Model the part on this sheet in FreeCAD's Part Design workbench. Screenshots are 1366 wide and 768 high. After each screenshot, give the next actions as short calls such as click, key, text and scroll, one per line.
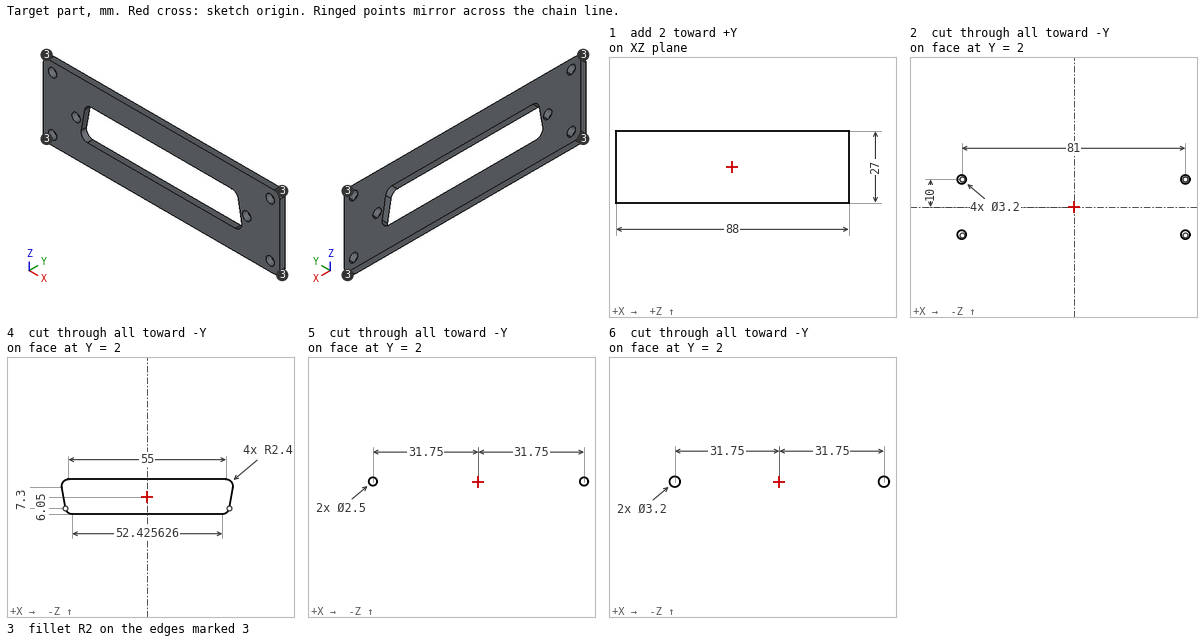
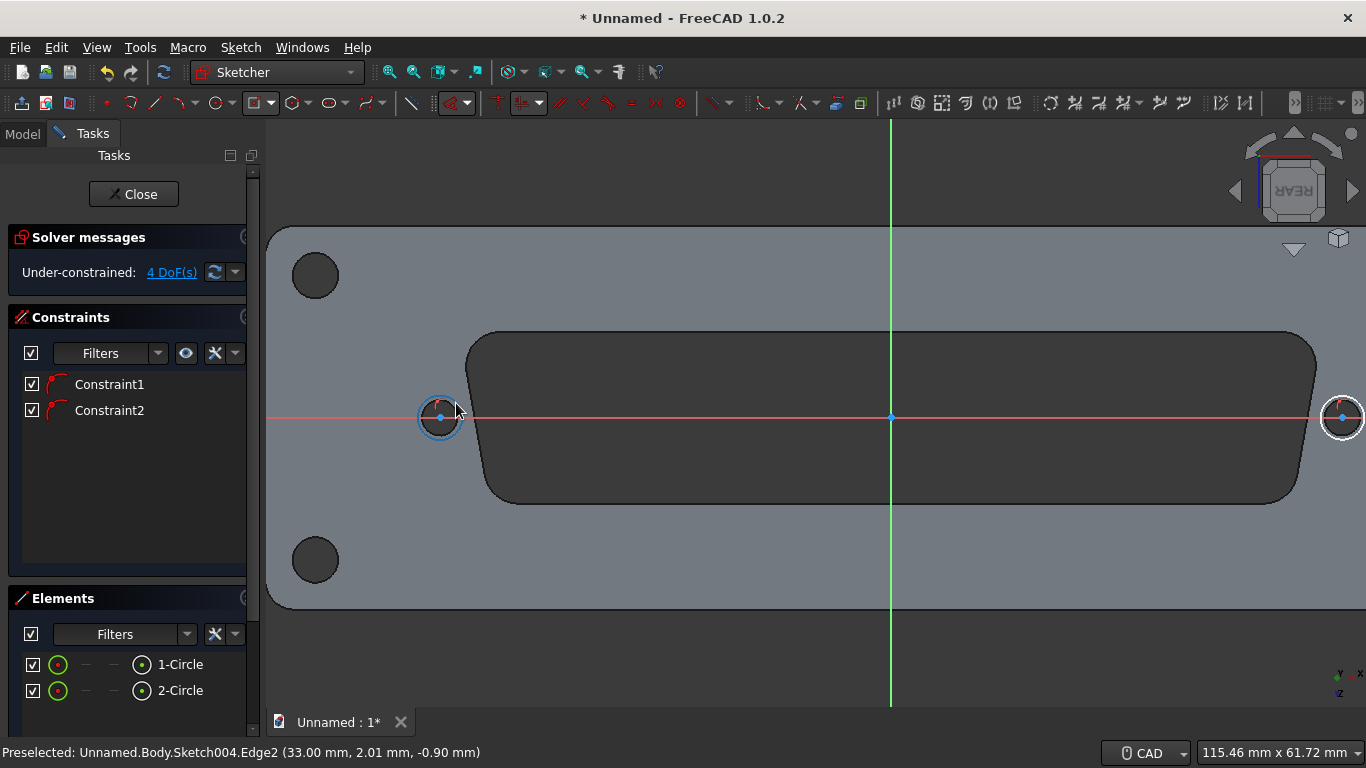
click(456, 402)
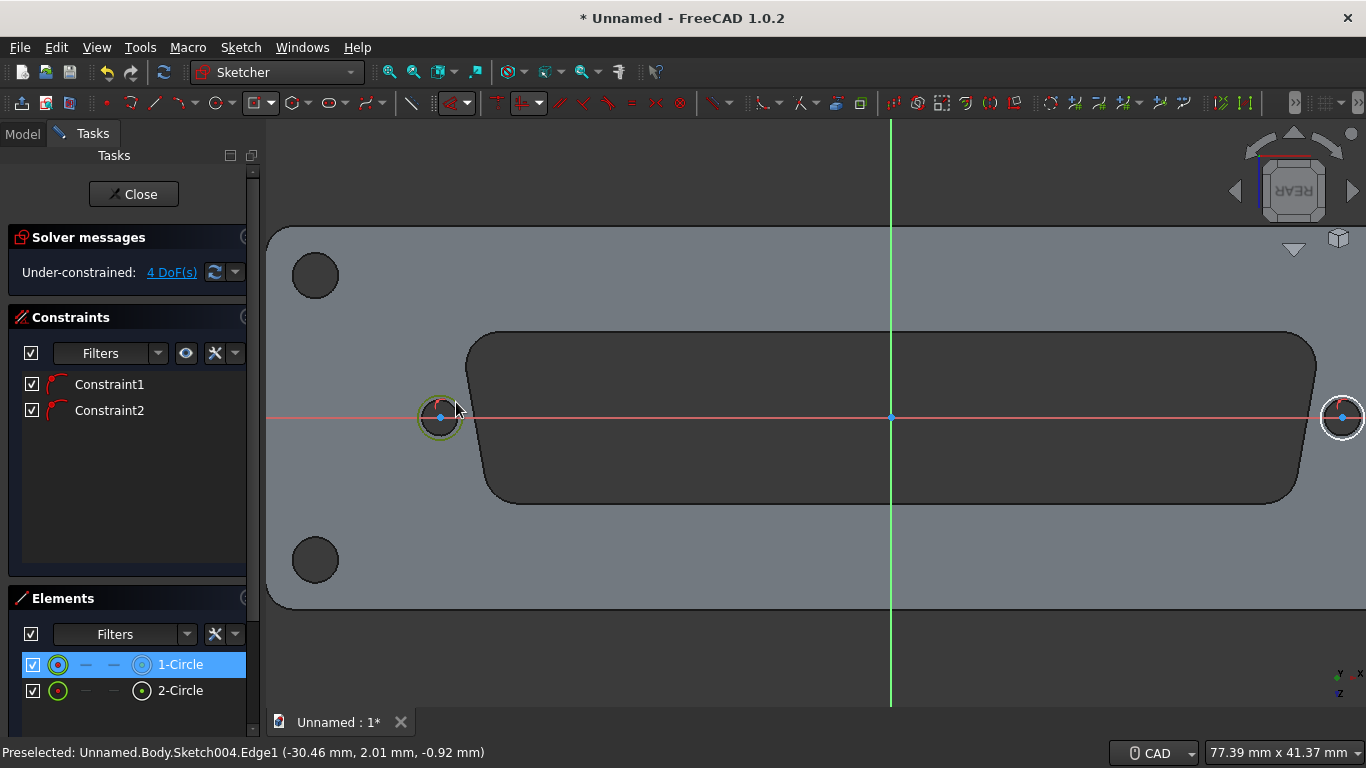
scroll(456, 403, down, 2)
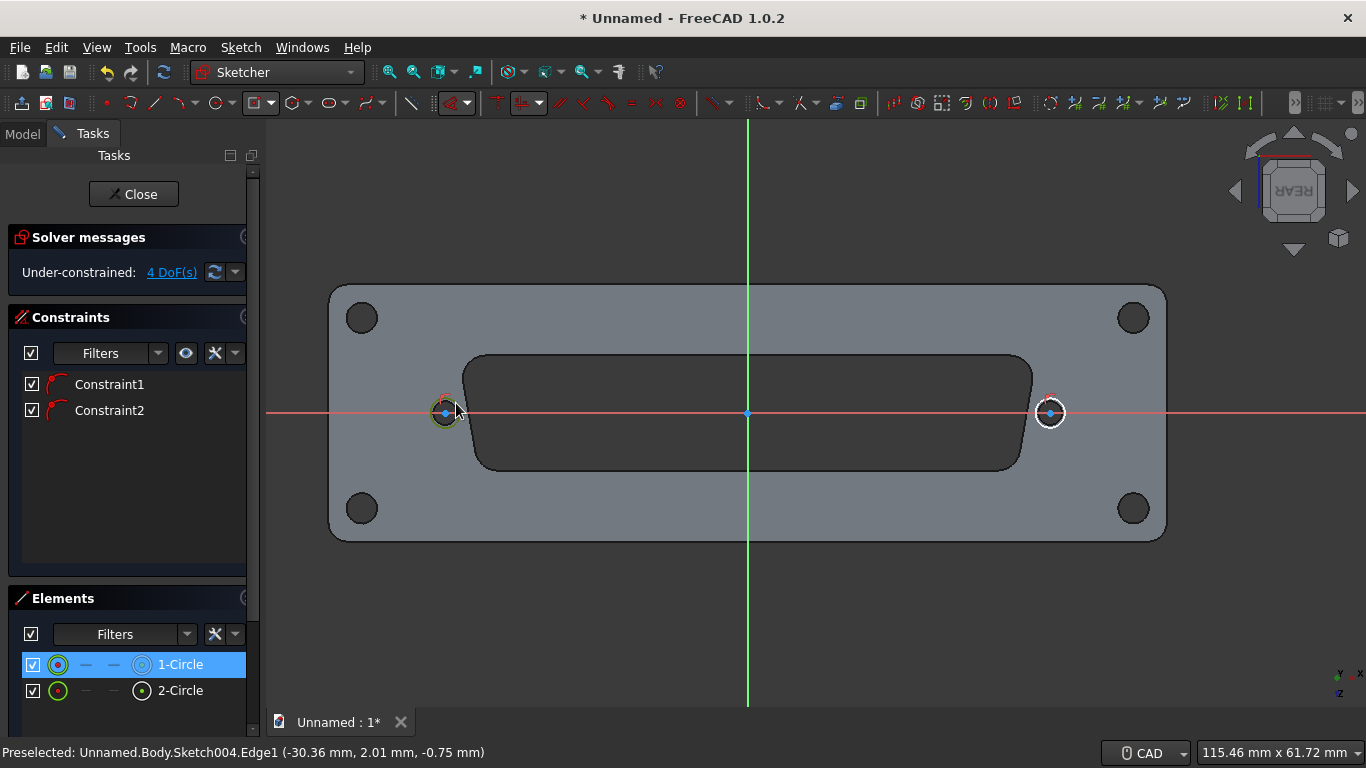
scroll(1061, 403, up, 2)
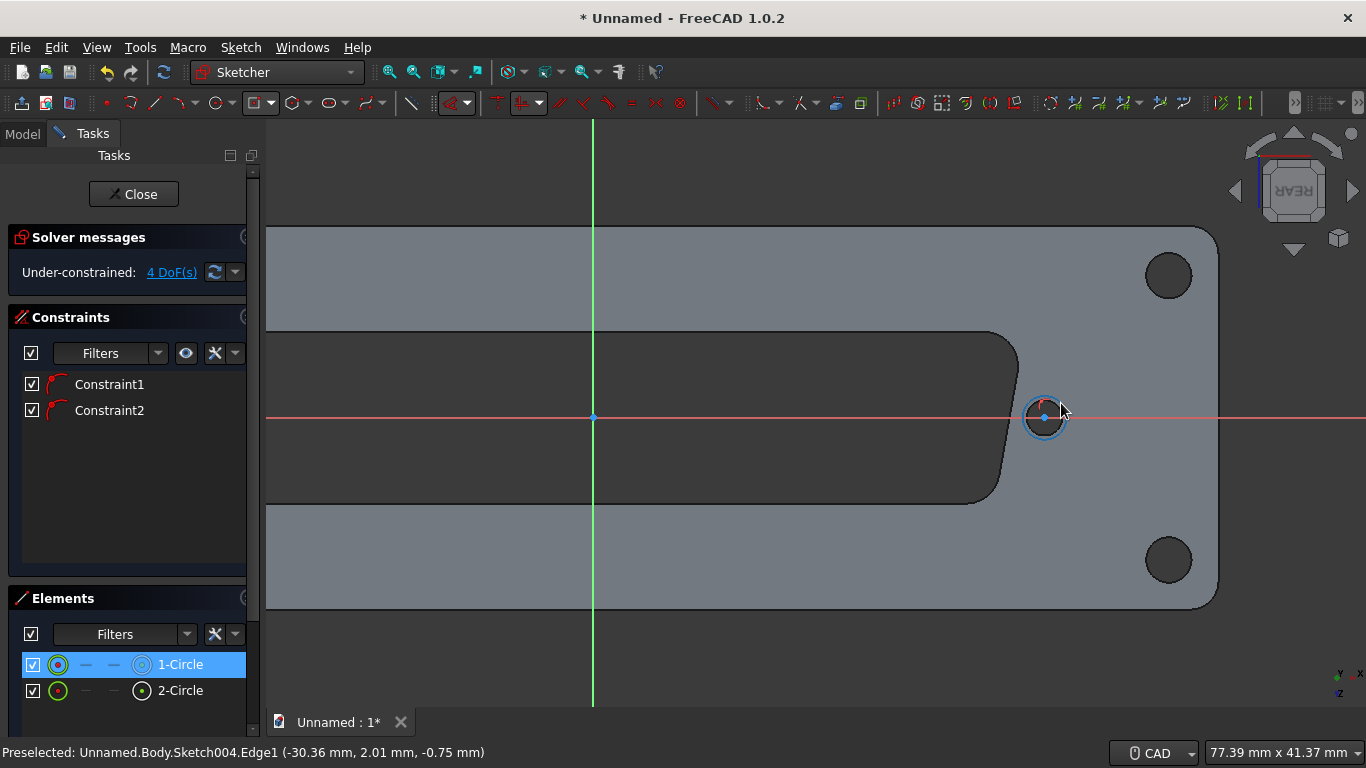
click(1060, 402)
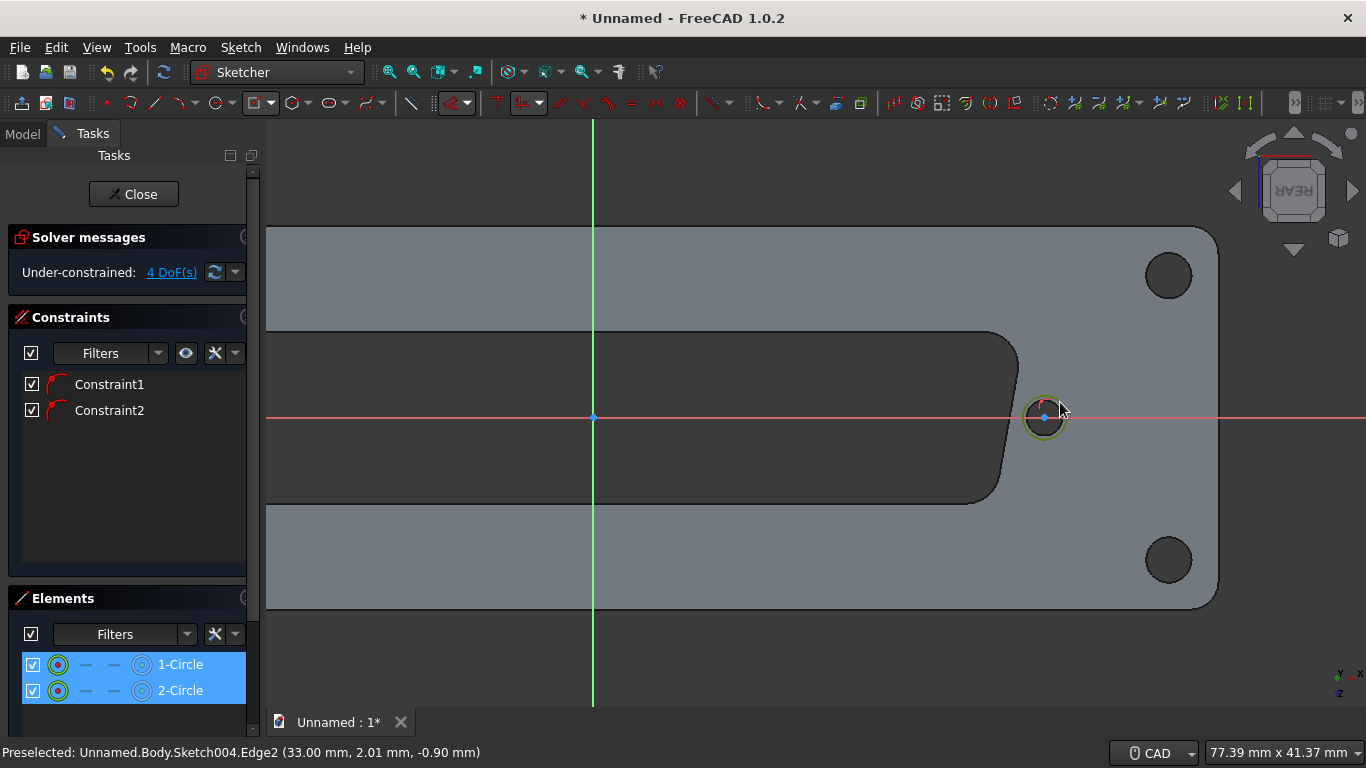
key(e)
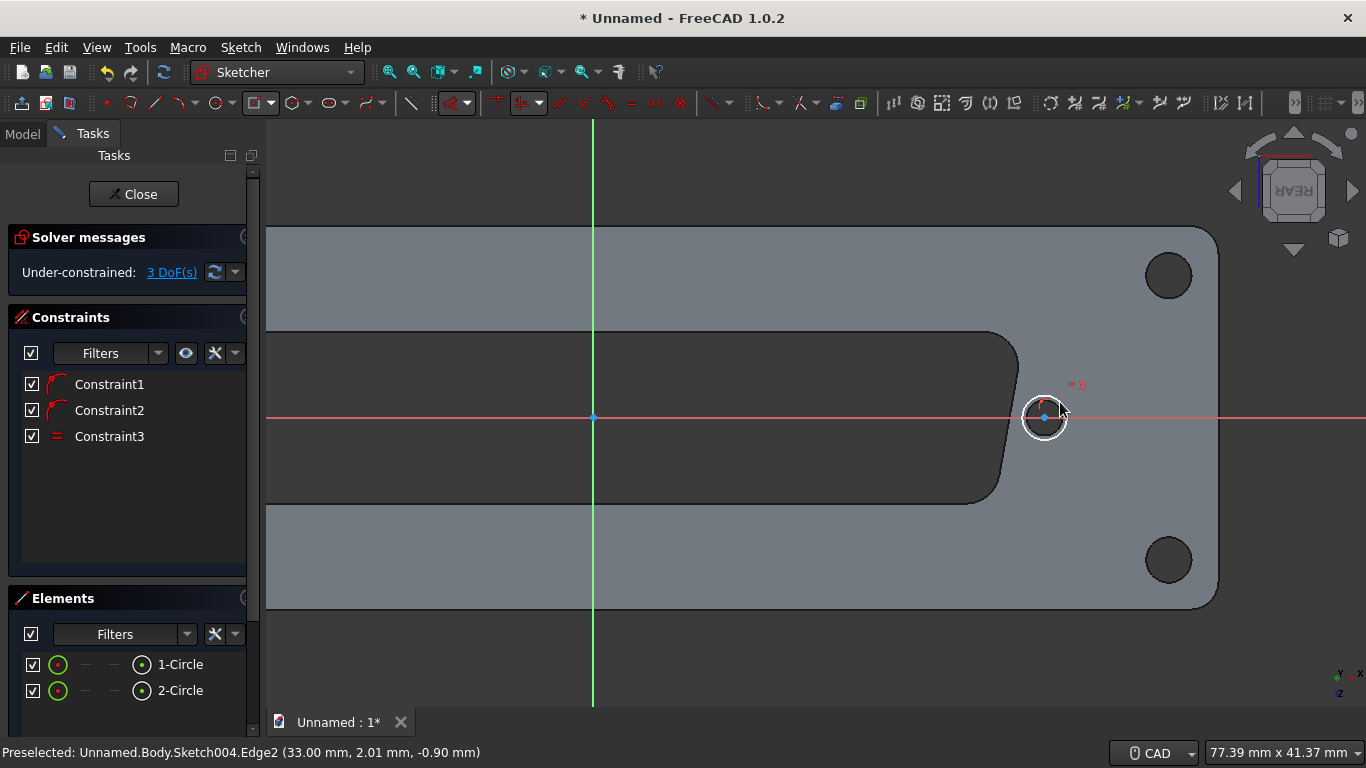
scroll(1061, 403, down, 2)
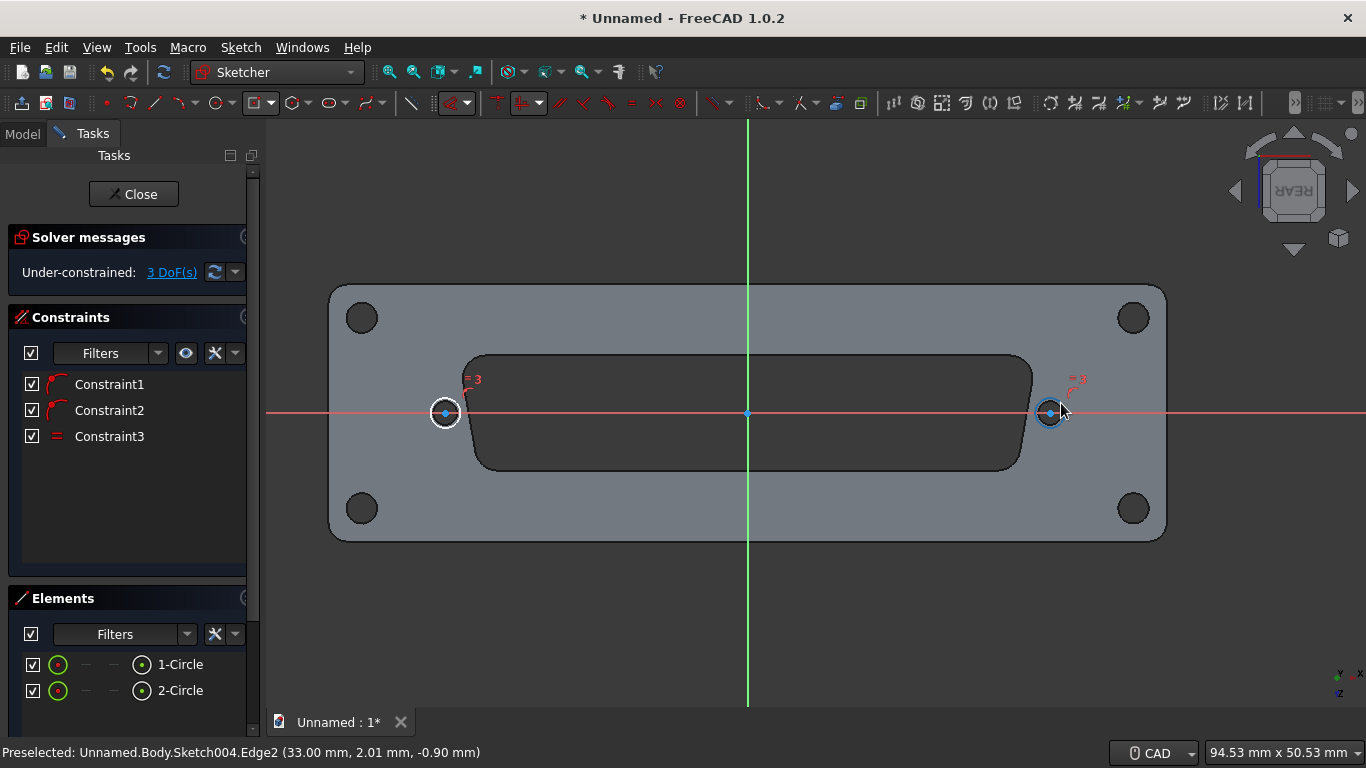
scroll(456, 403, up, 2)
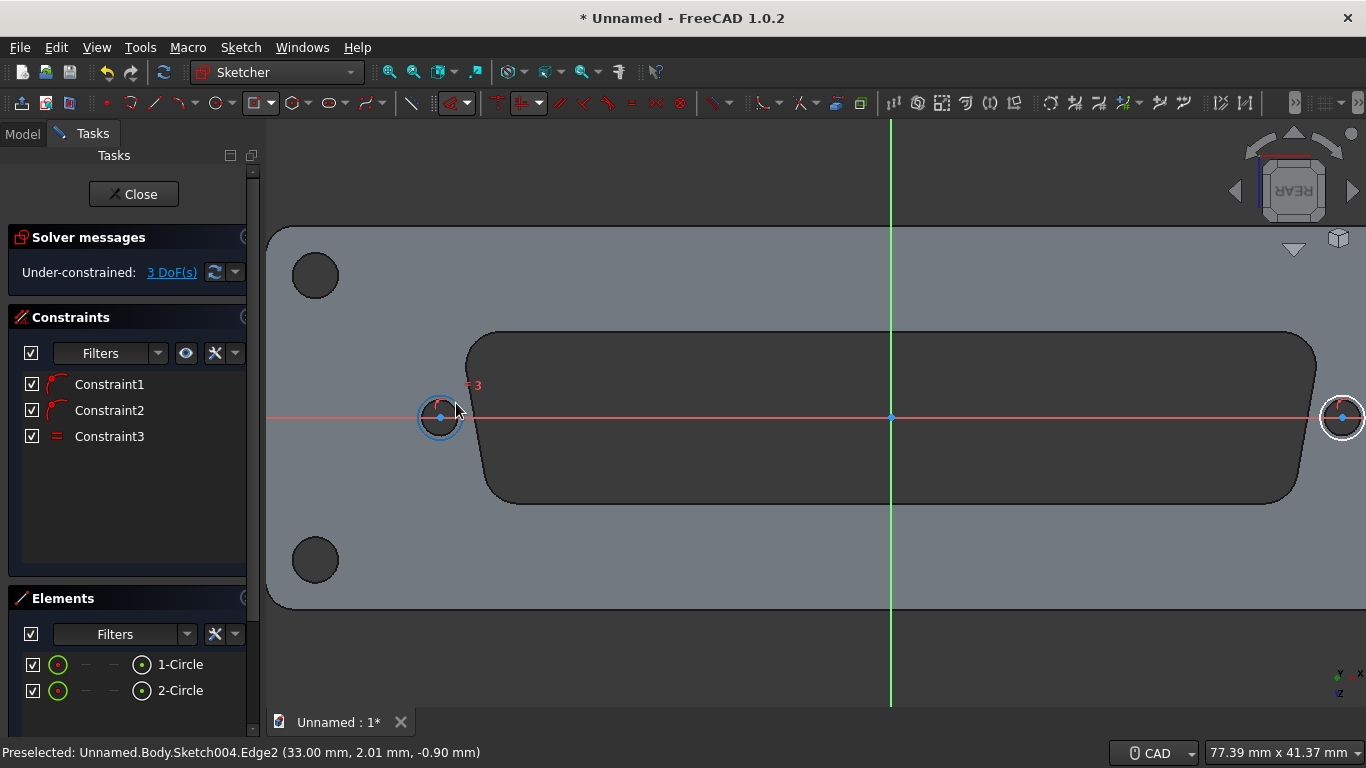
click(456, 402)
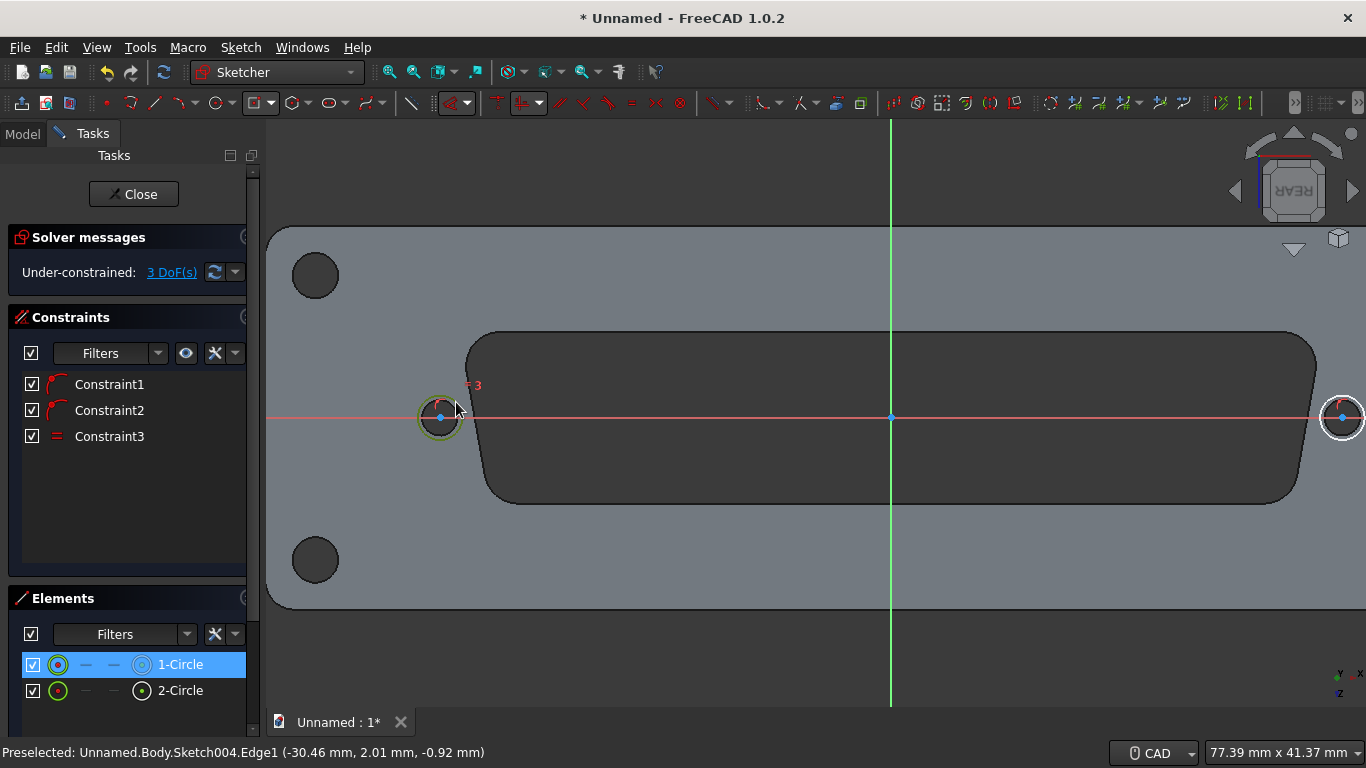
key(k)
key(o)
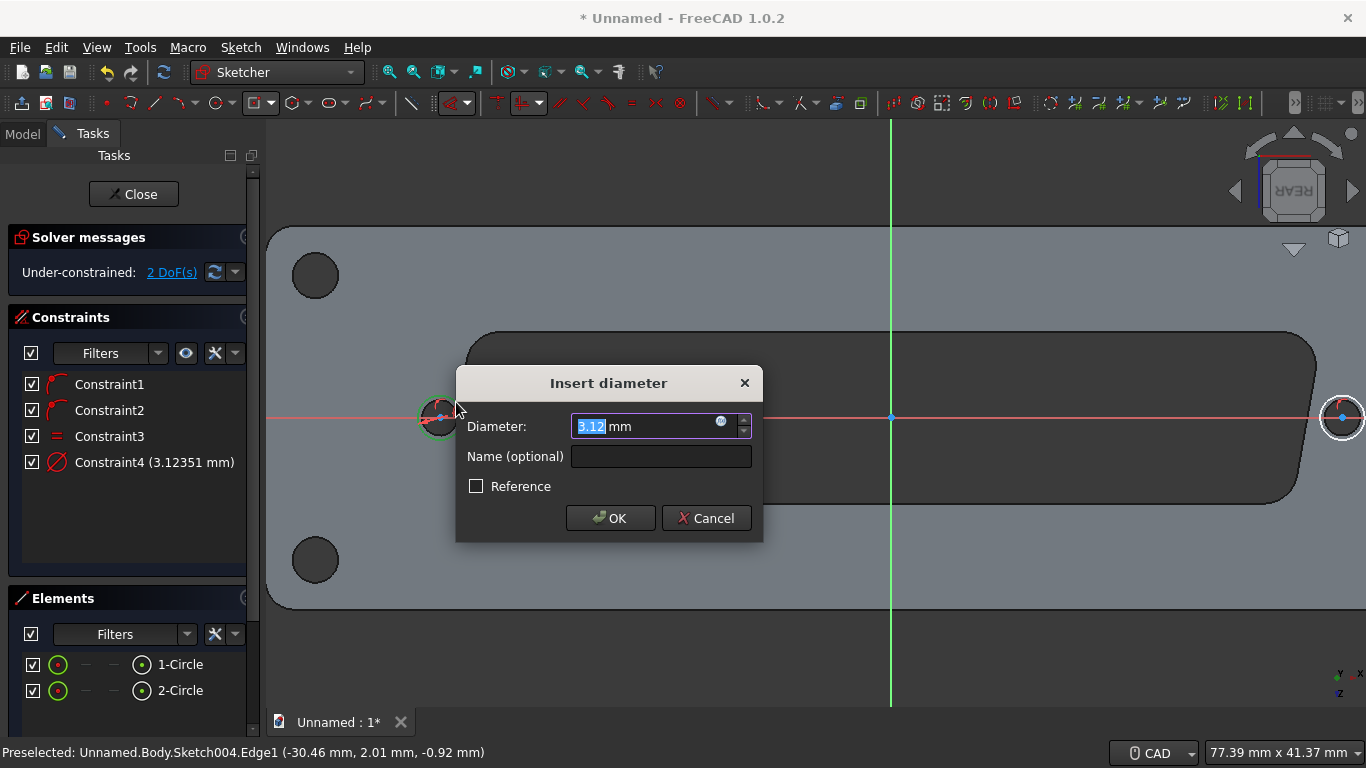
text(3.2)
key(Return)